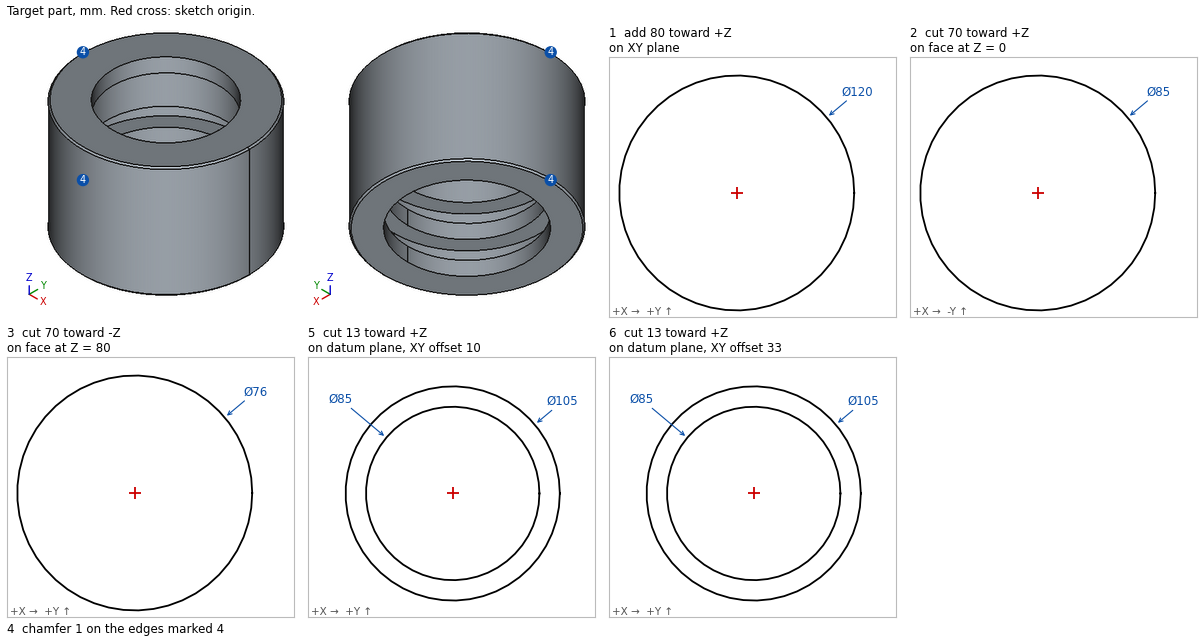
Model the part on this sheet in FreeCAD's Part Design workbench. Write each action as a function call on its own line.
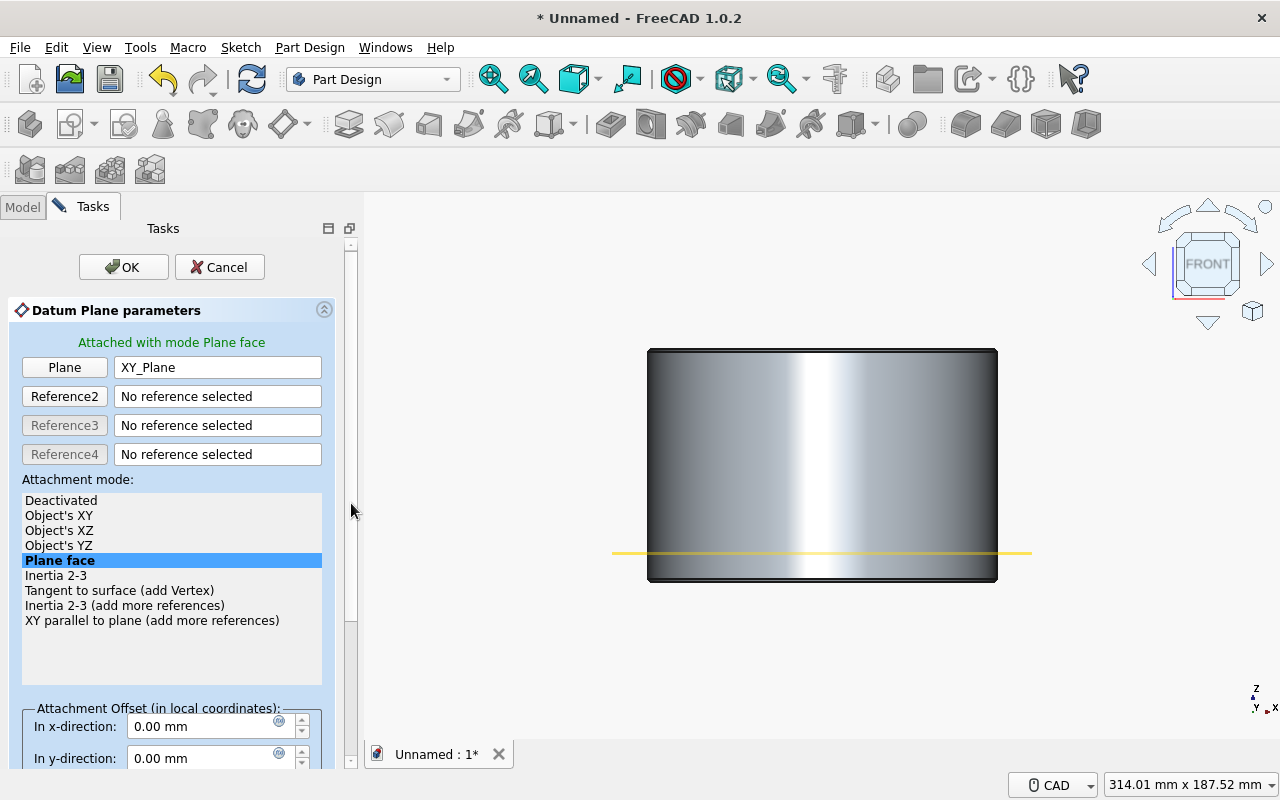
click(124, 267)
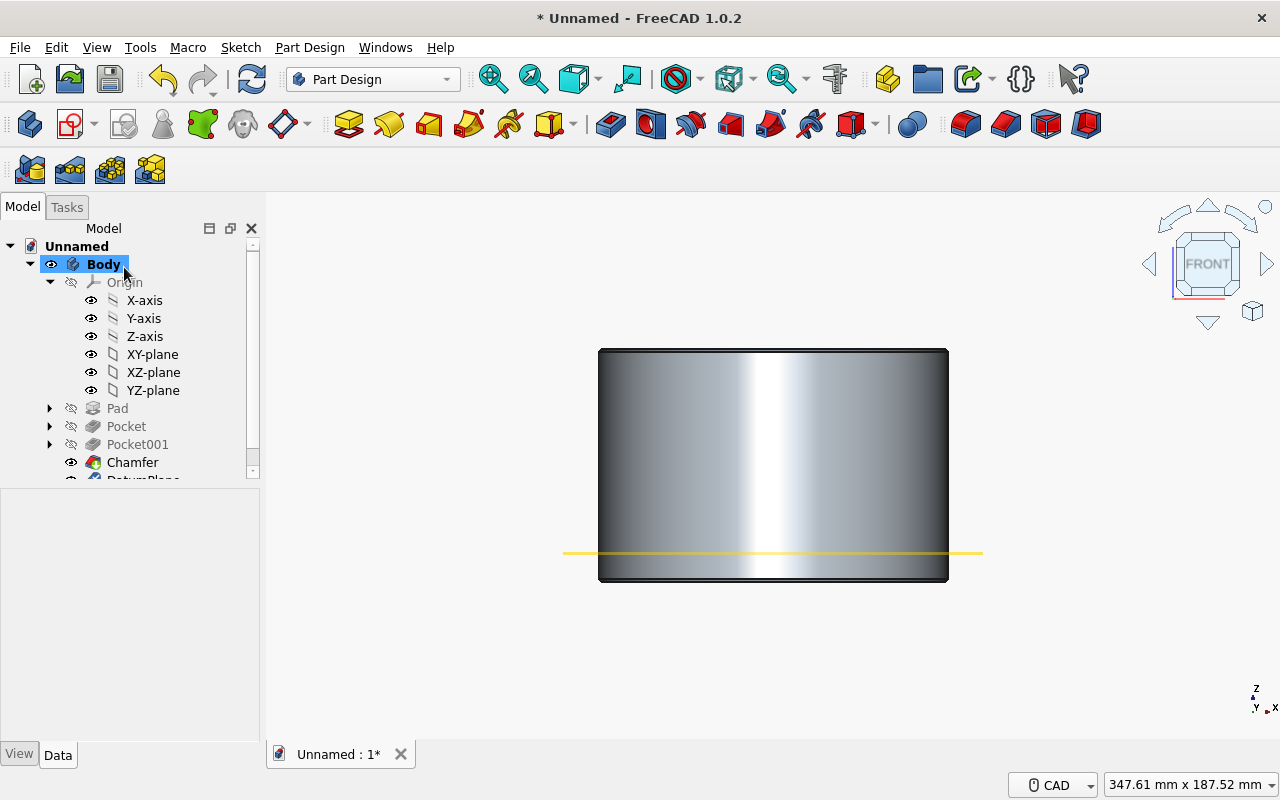
scroll(100, 350, down, 3)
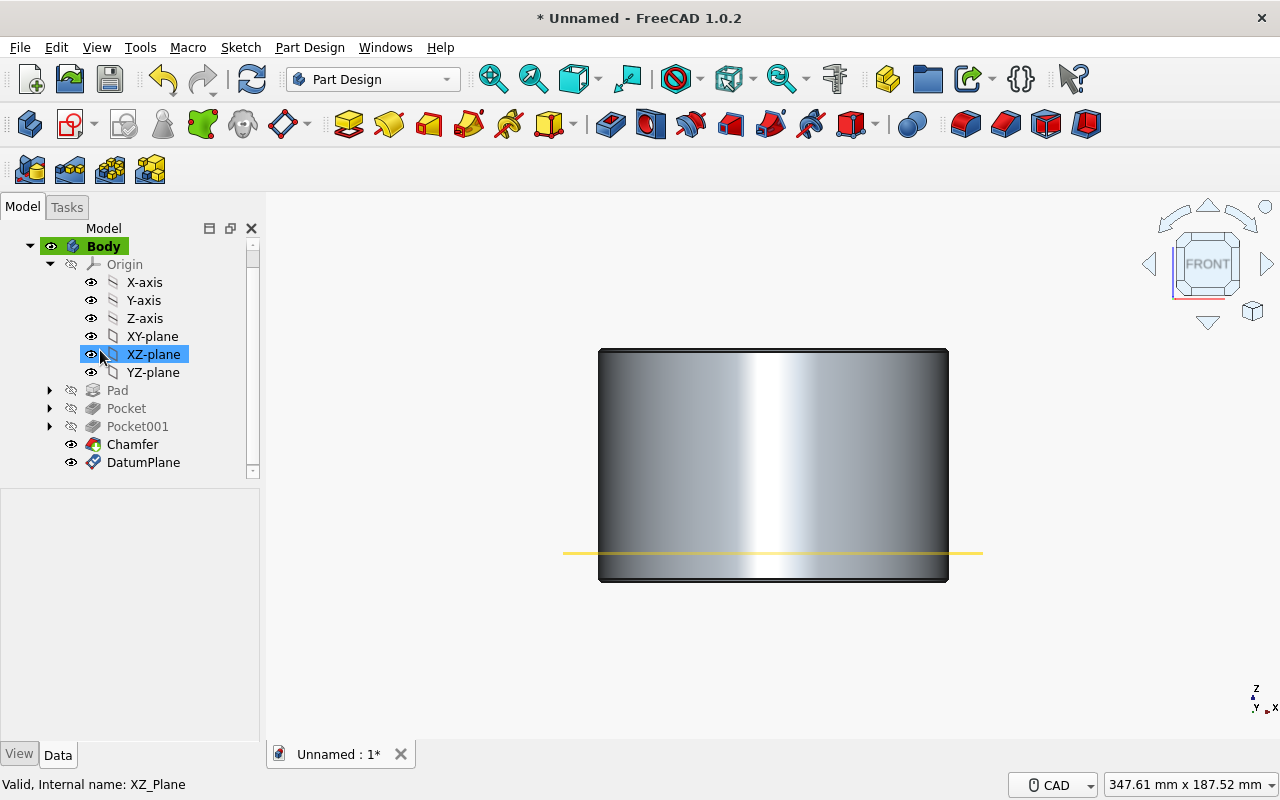
click(116, 462)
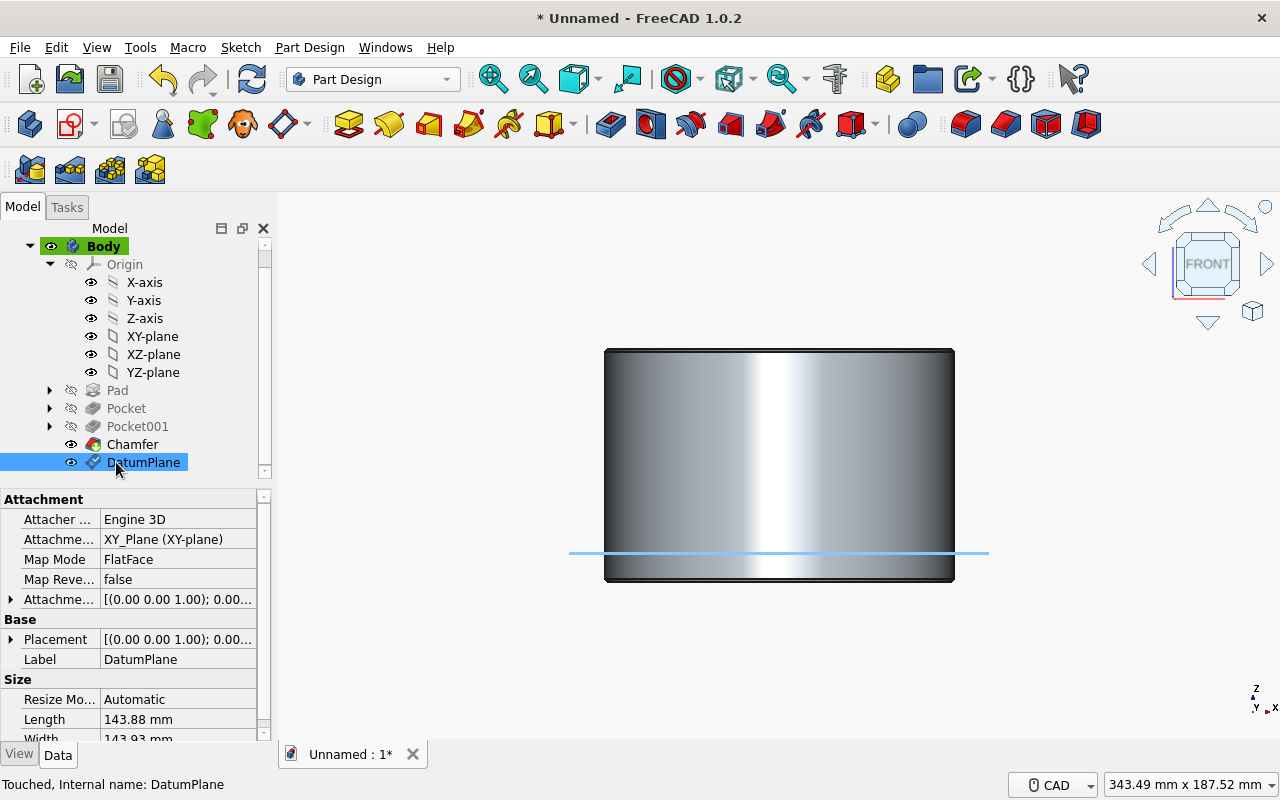
click(70, 124)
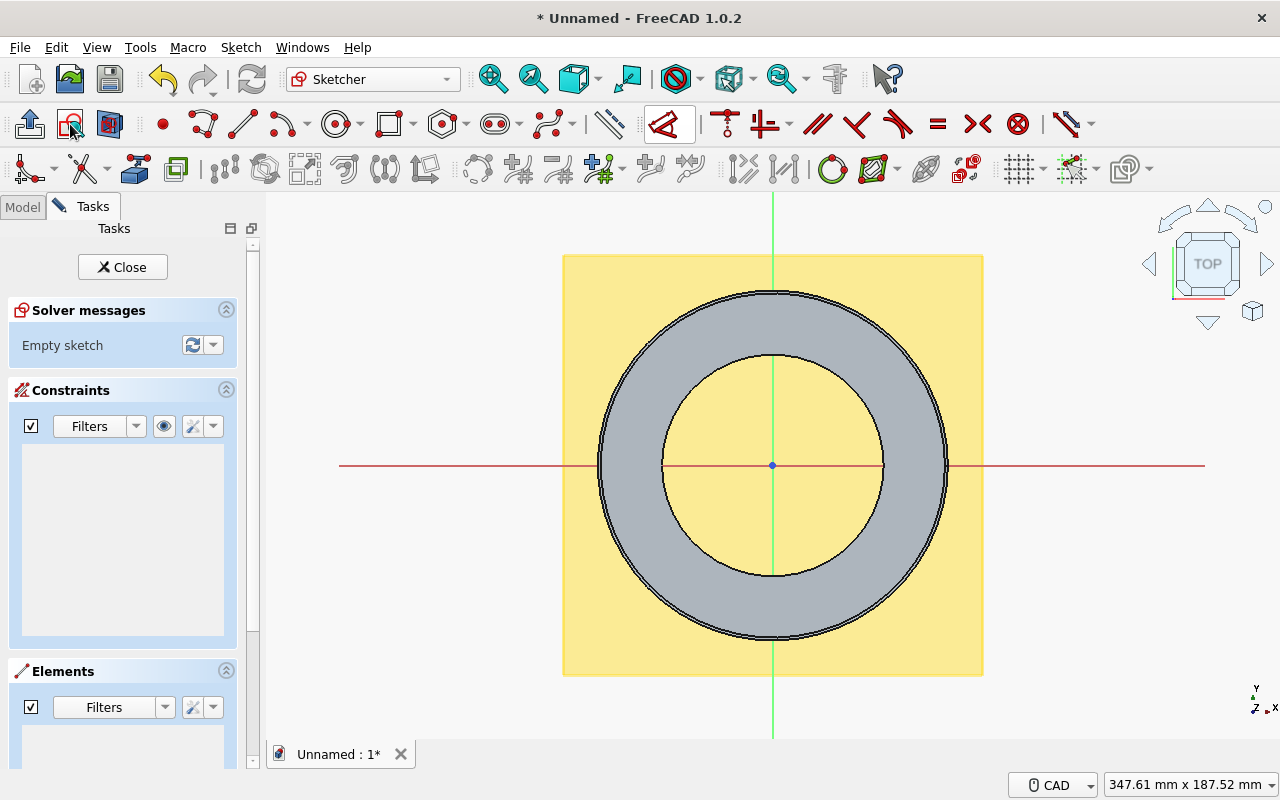
click(110, 124)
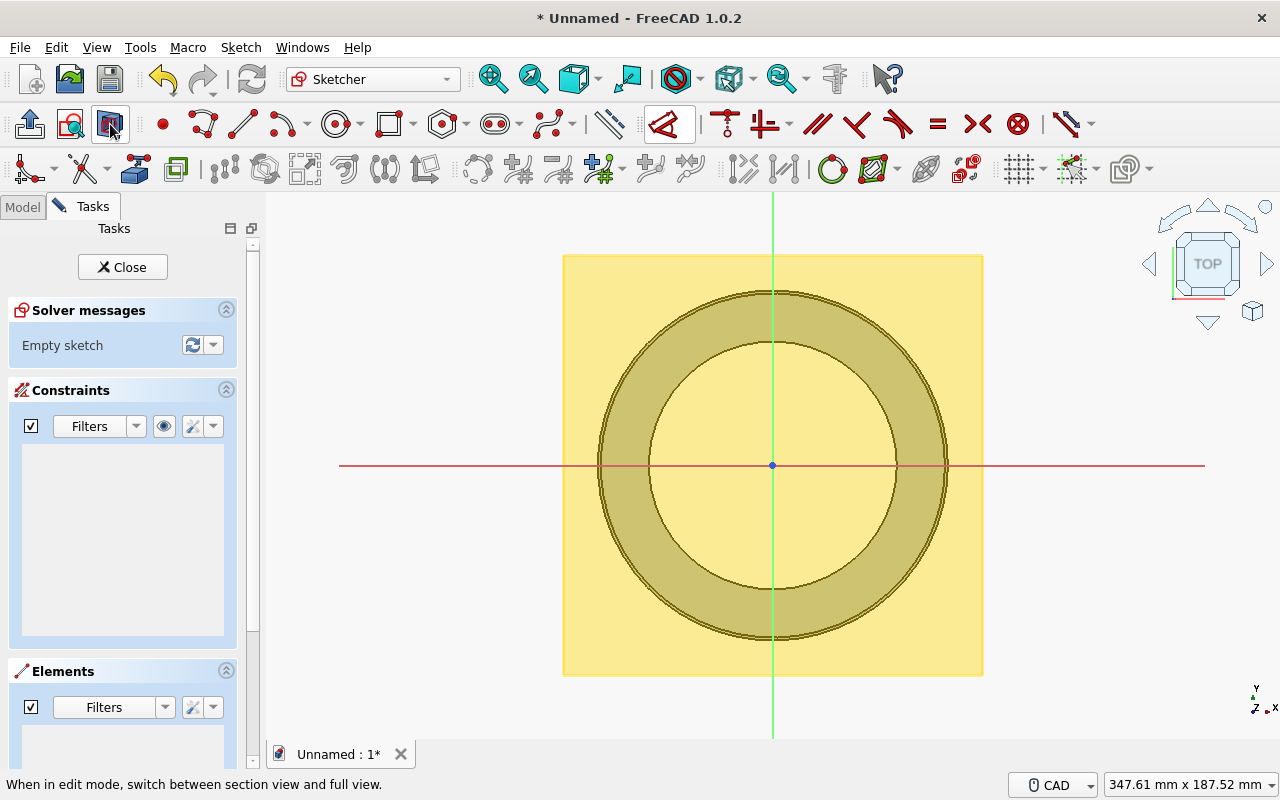
click(336, 124)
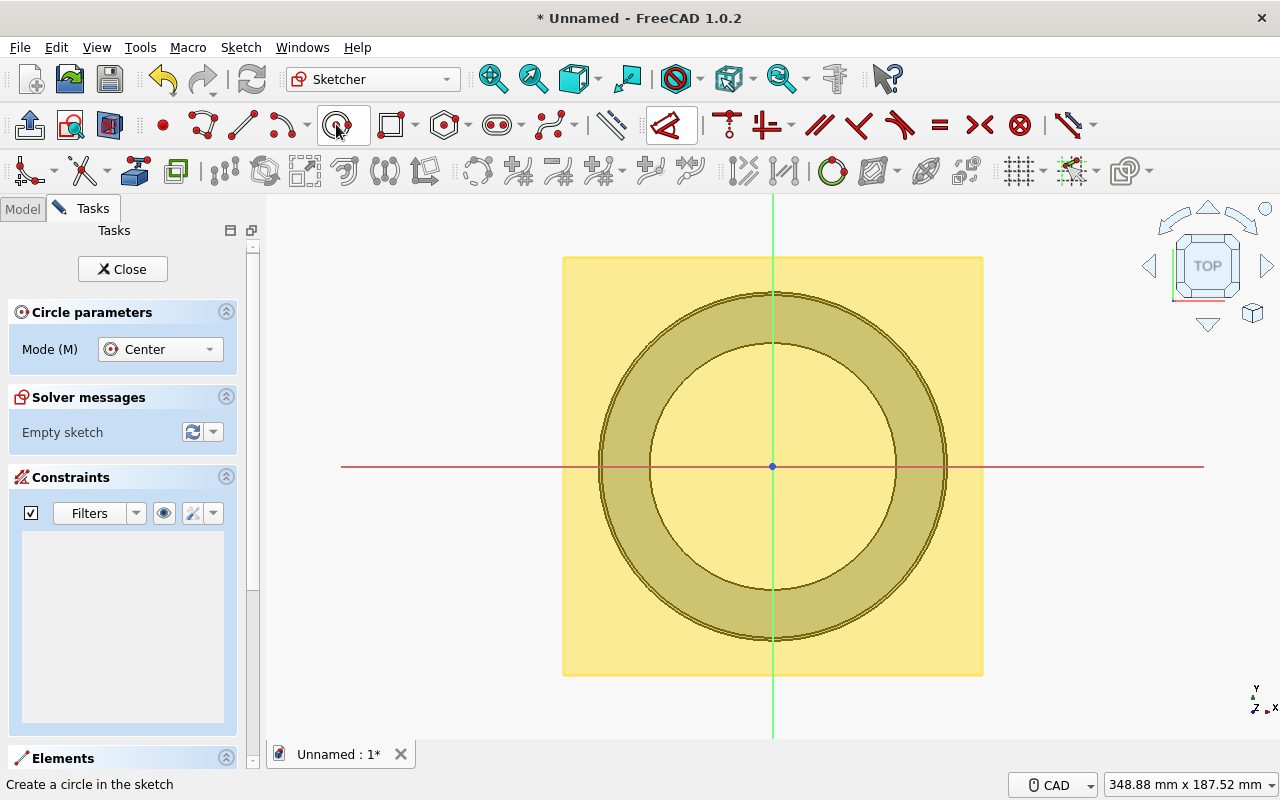
click(773, 466)
click(881, 359)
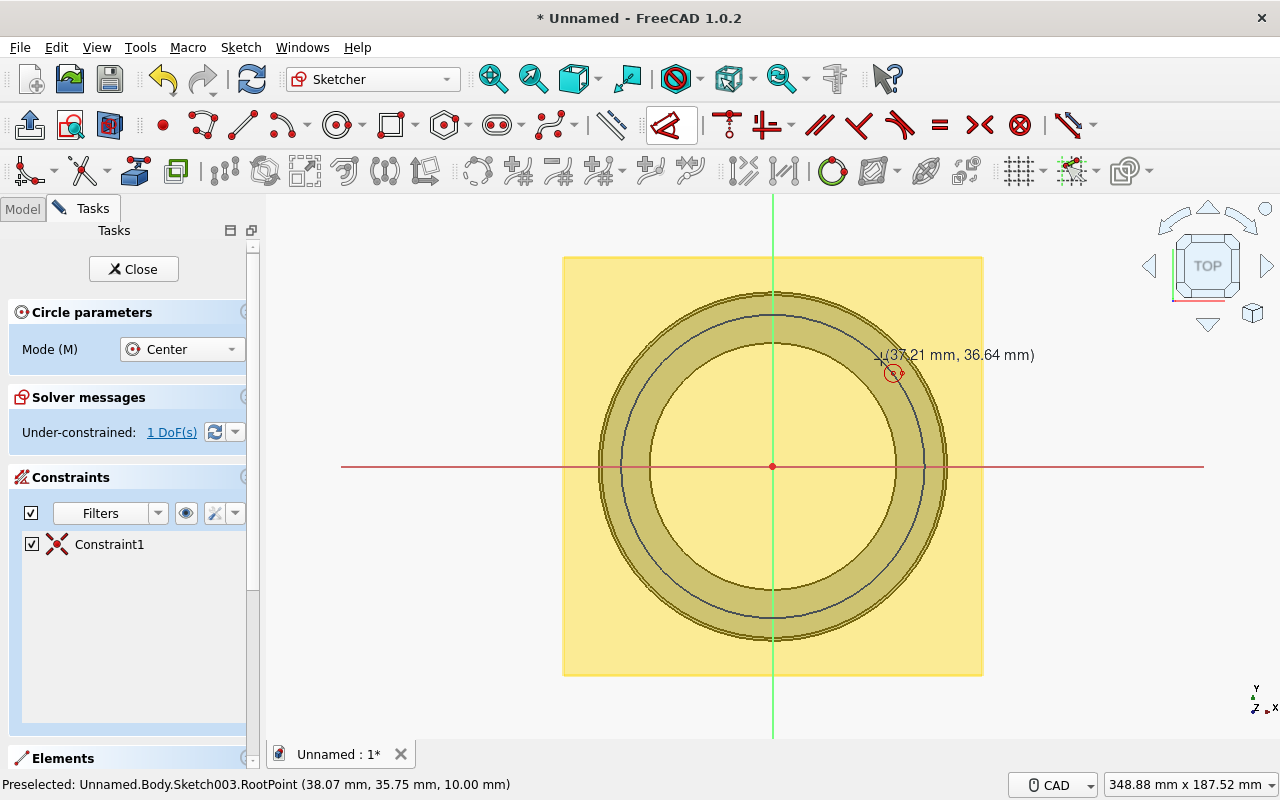
click(773, 466)
click(860, 379)
key(Escape)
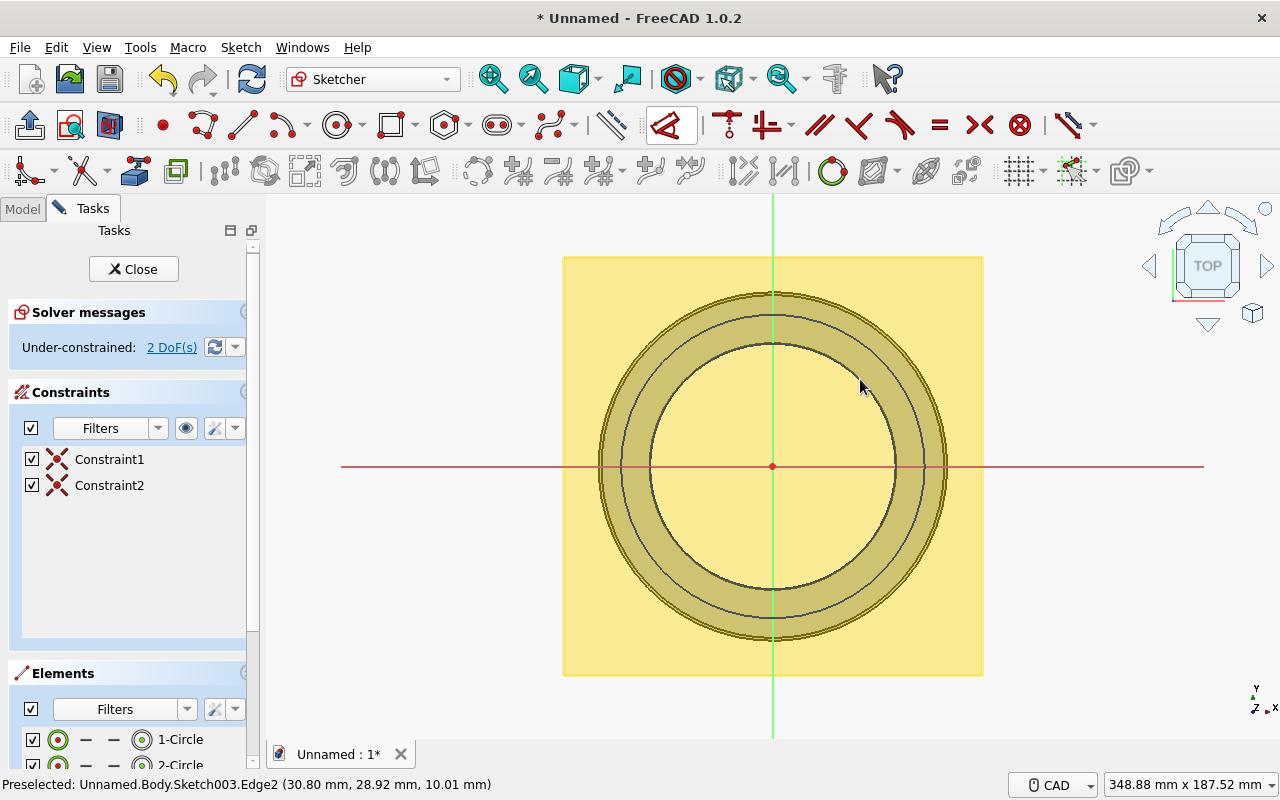
click(880, 359)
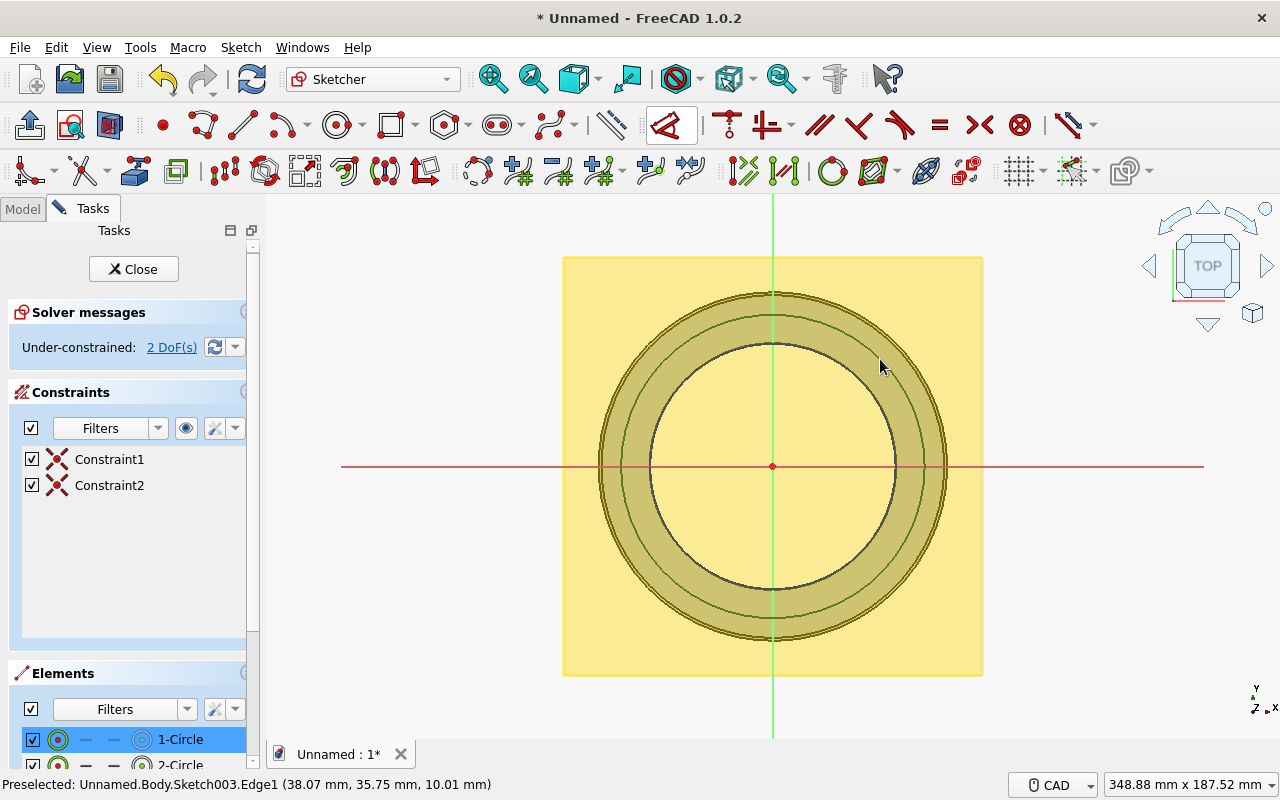
click(692, 126)